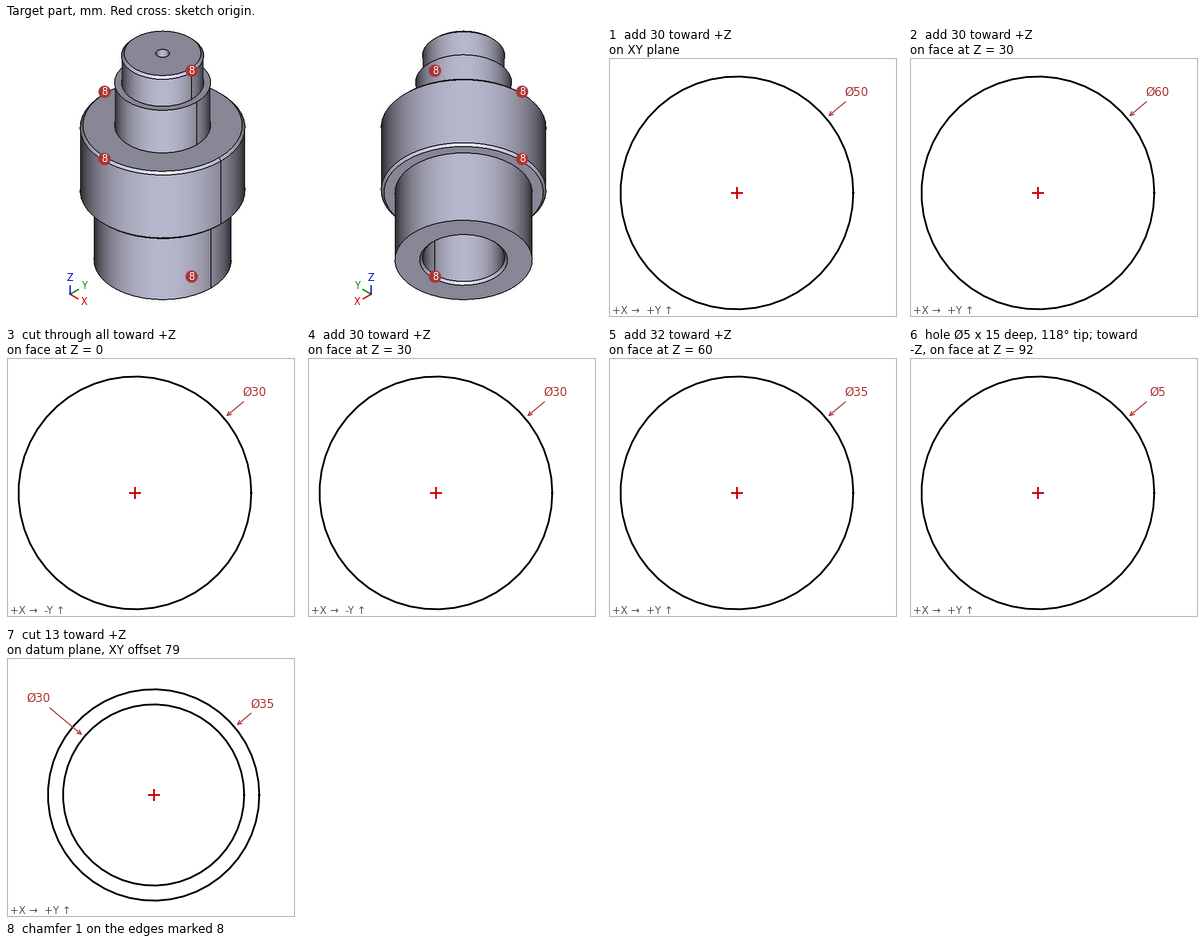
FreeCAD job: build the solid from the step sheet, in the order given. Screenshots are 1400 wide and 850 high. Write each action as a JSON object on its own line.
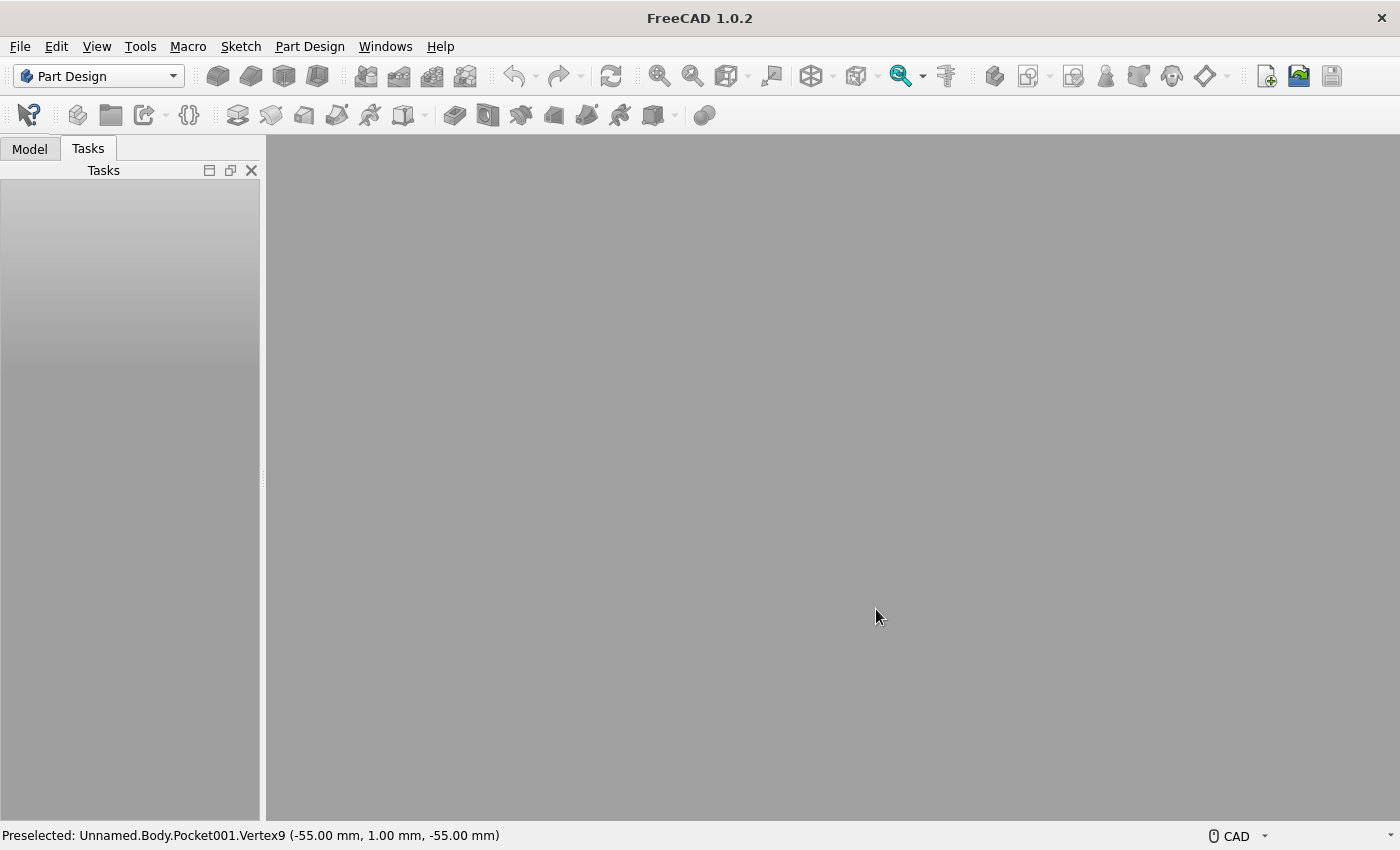
{"action": "key", "text": "ctrl+n"}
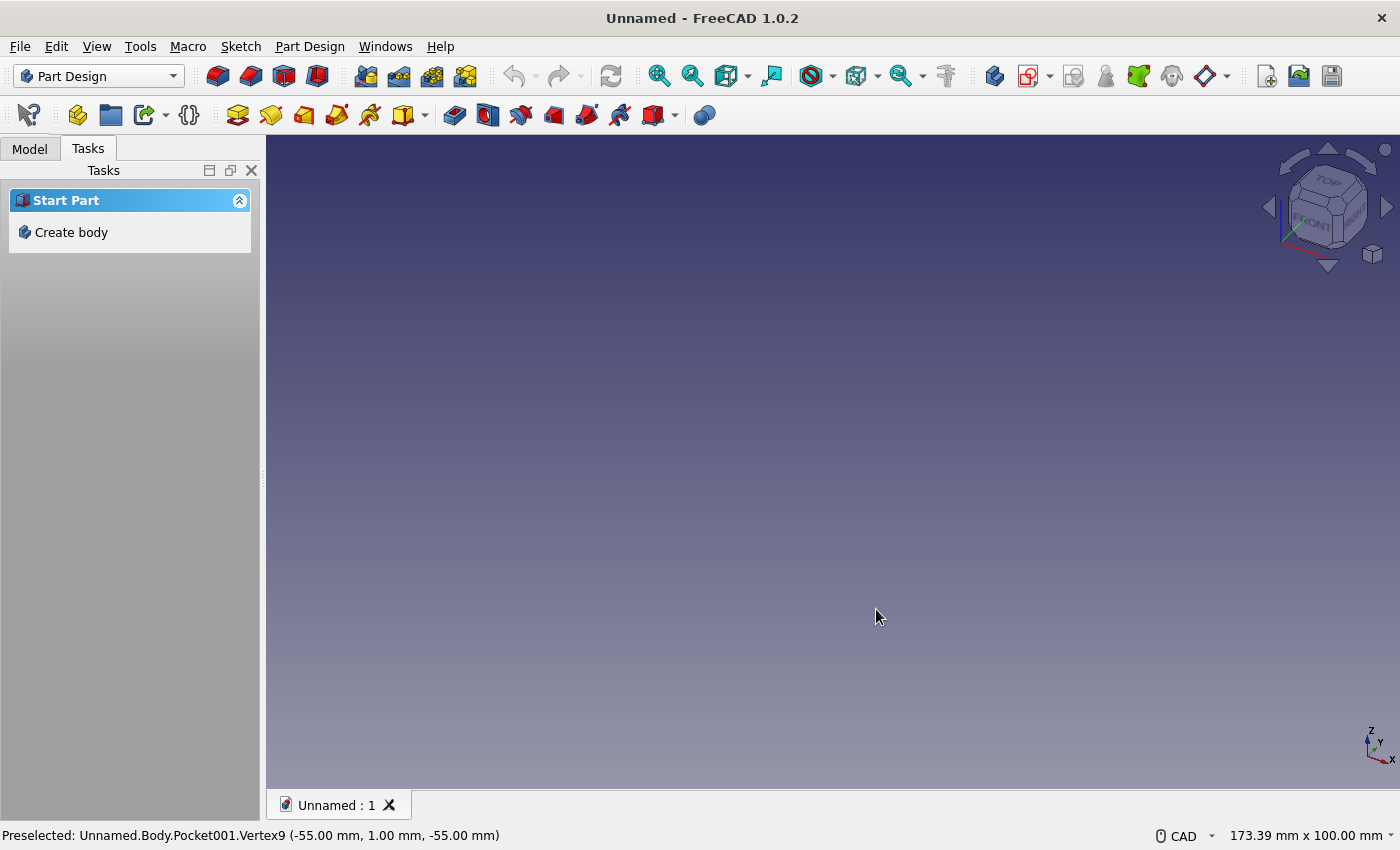
{"action": "left_click", "coordinate": [1028, 76]}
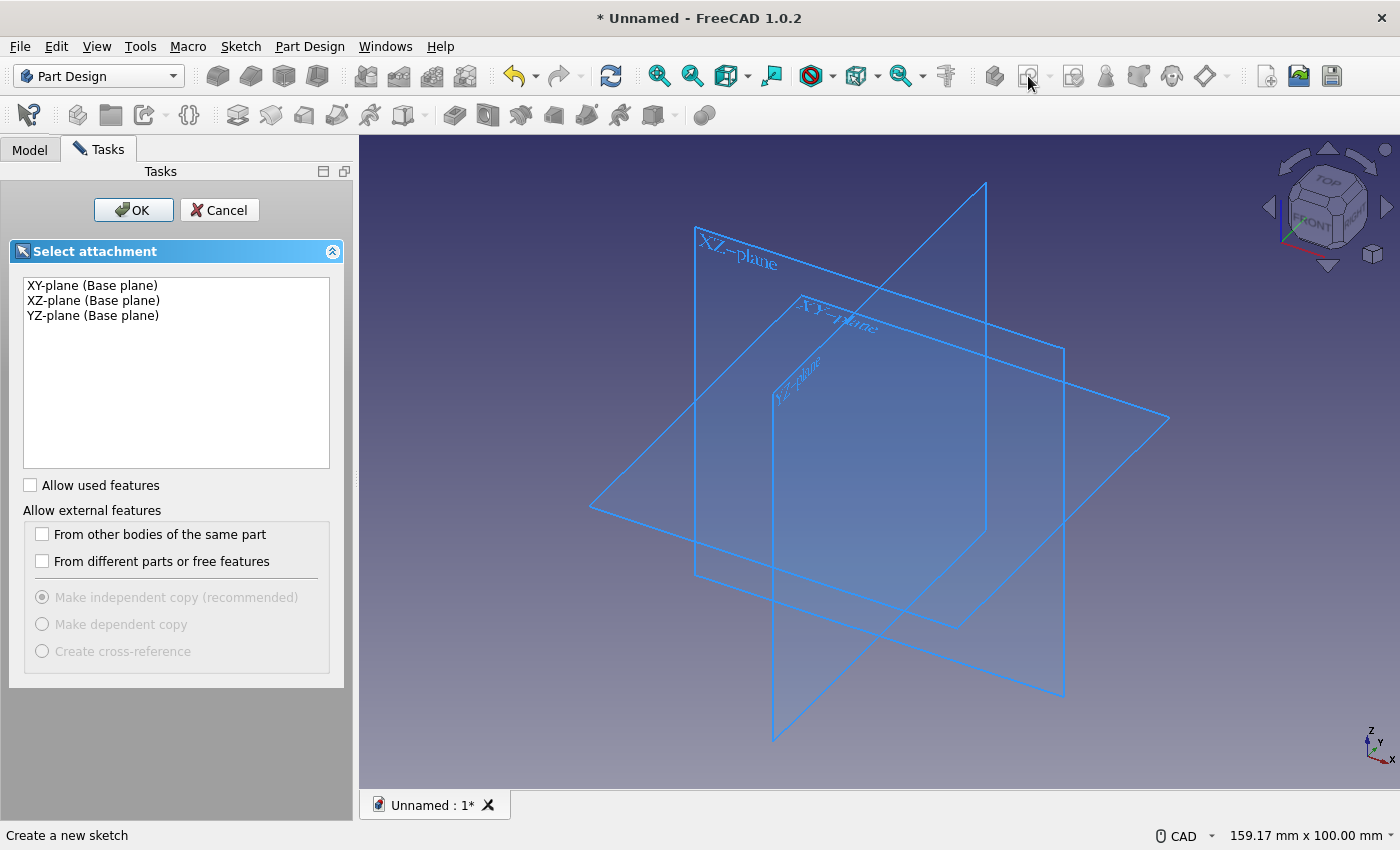
{"action": "left_click", "coordinate": [84, 286]}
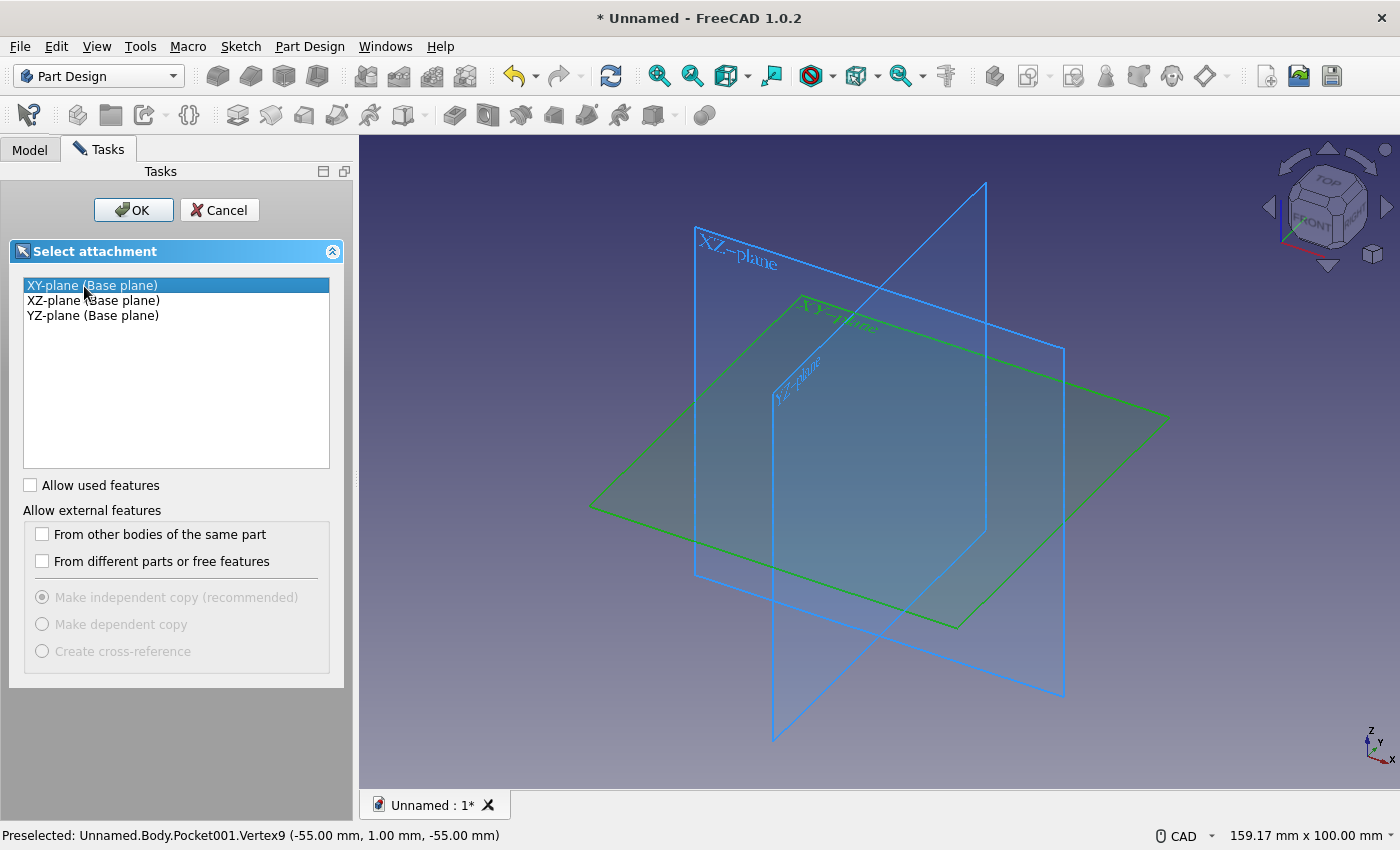
{"action": "left_click", "coordinate": [134, 210]}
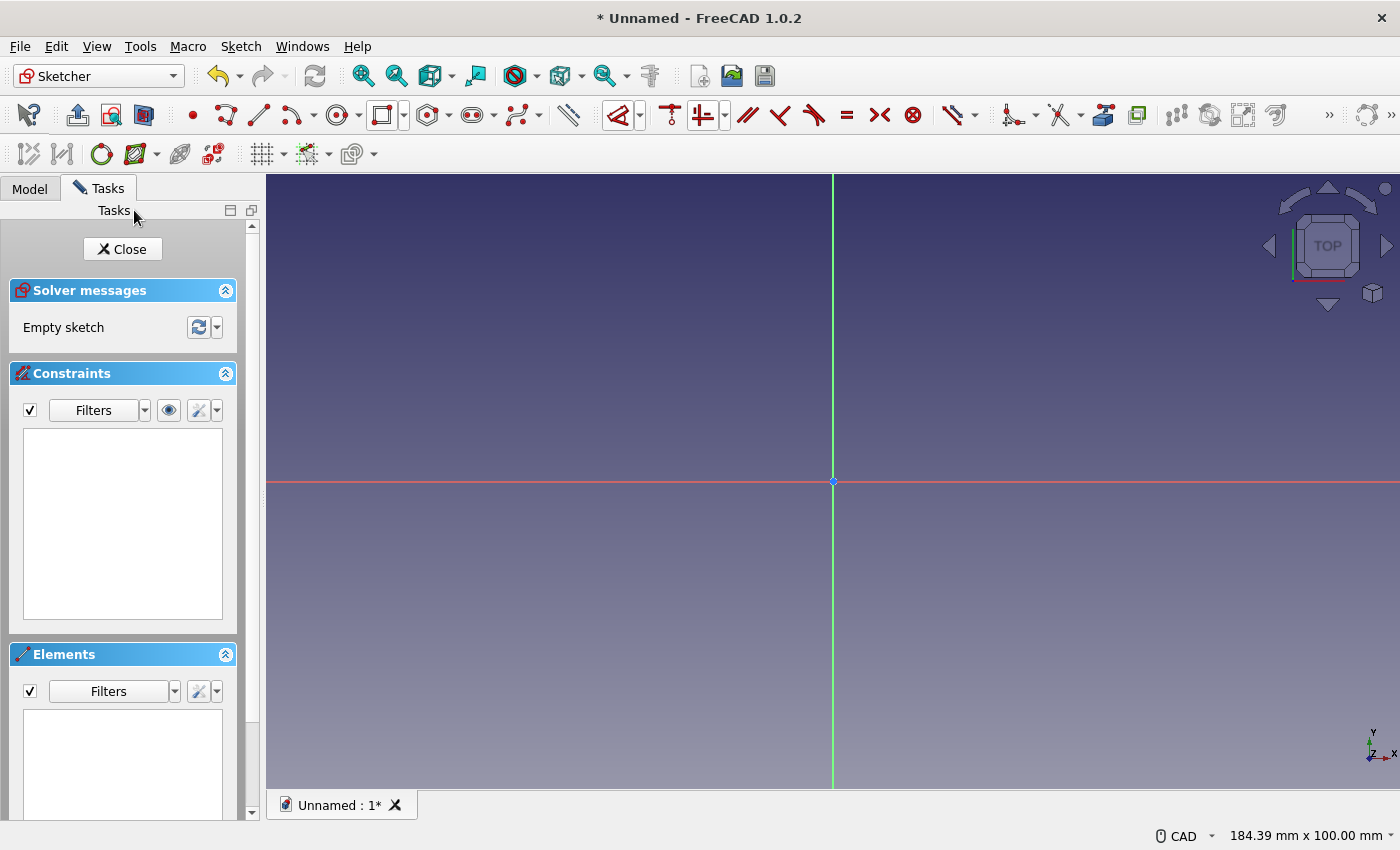
{"action": "left_click", "coordinate": [336, 116]}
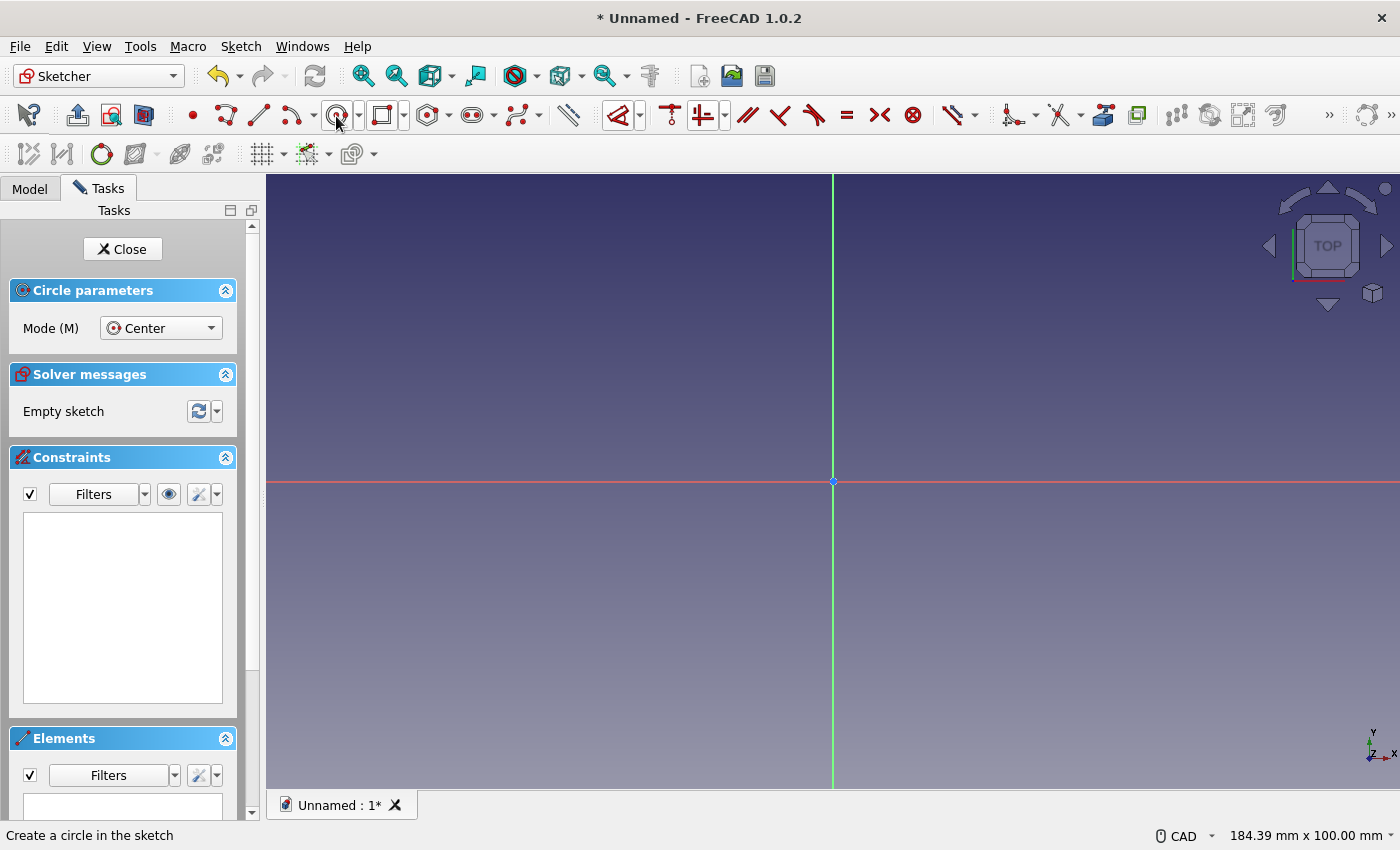
{"action": "left_click", "coordinate": [833, 482]}
{"action": "left_click", "coordinate": [942, 373]}
{"action": "key", "text": "Escape"}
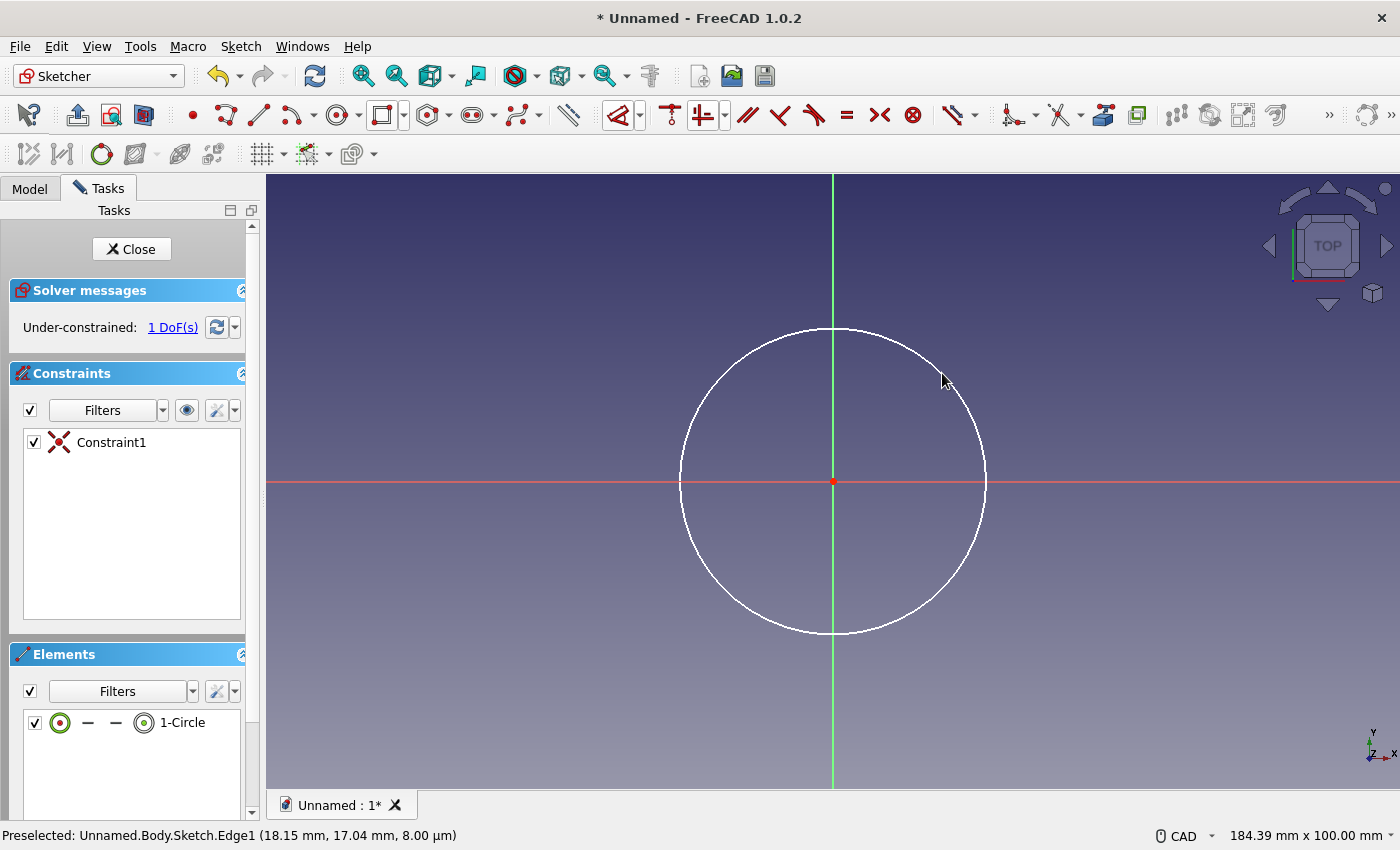
{"action": "left_click", "coordinate": [618, 116]}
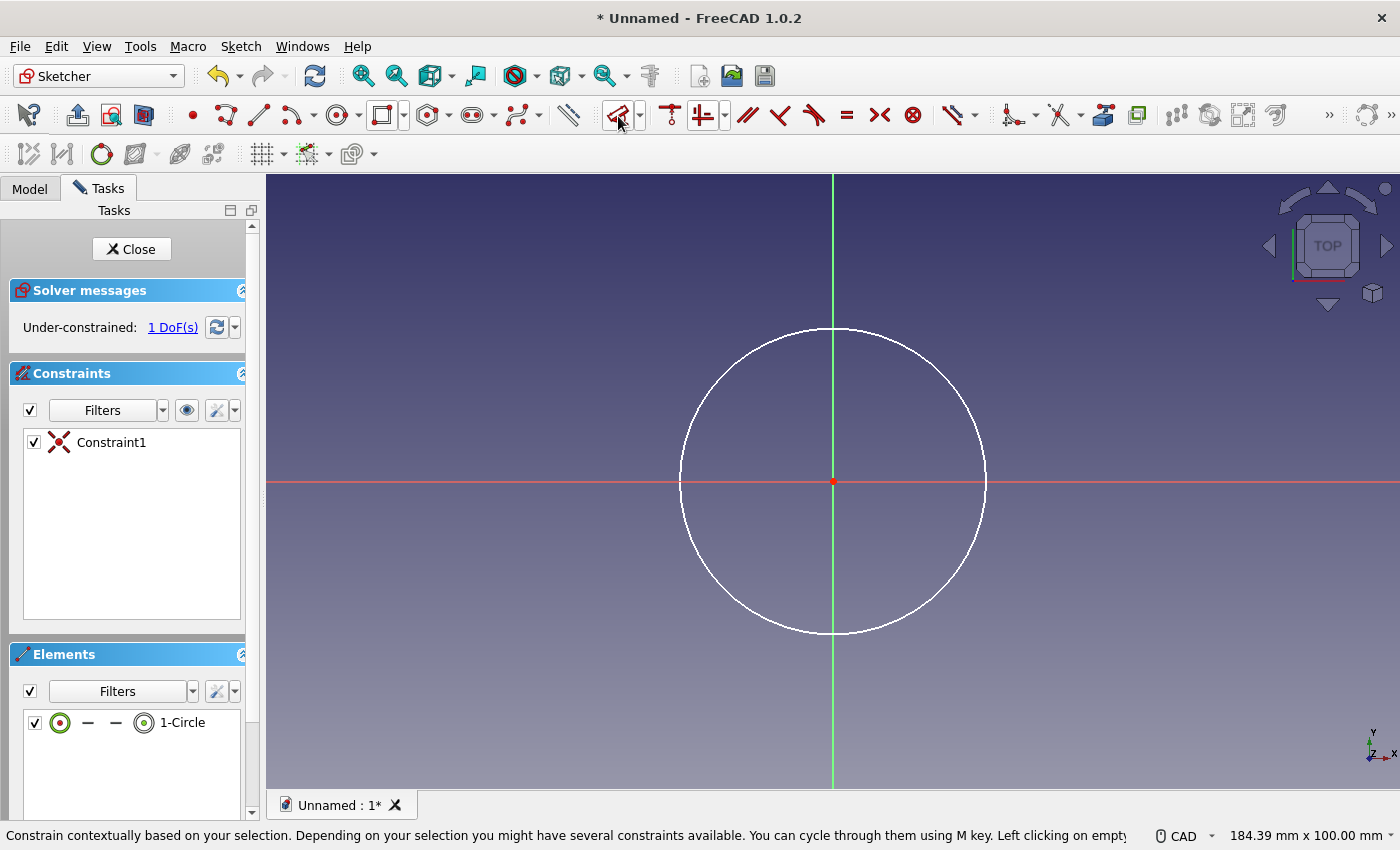
{"action": "left_click", "coordinate": [941, 373]}
{"action": "left_click", "coordinate": [964, 350]}